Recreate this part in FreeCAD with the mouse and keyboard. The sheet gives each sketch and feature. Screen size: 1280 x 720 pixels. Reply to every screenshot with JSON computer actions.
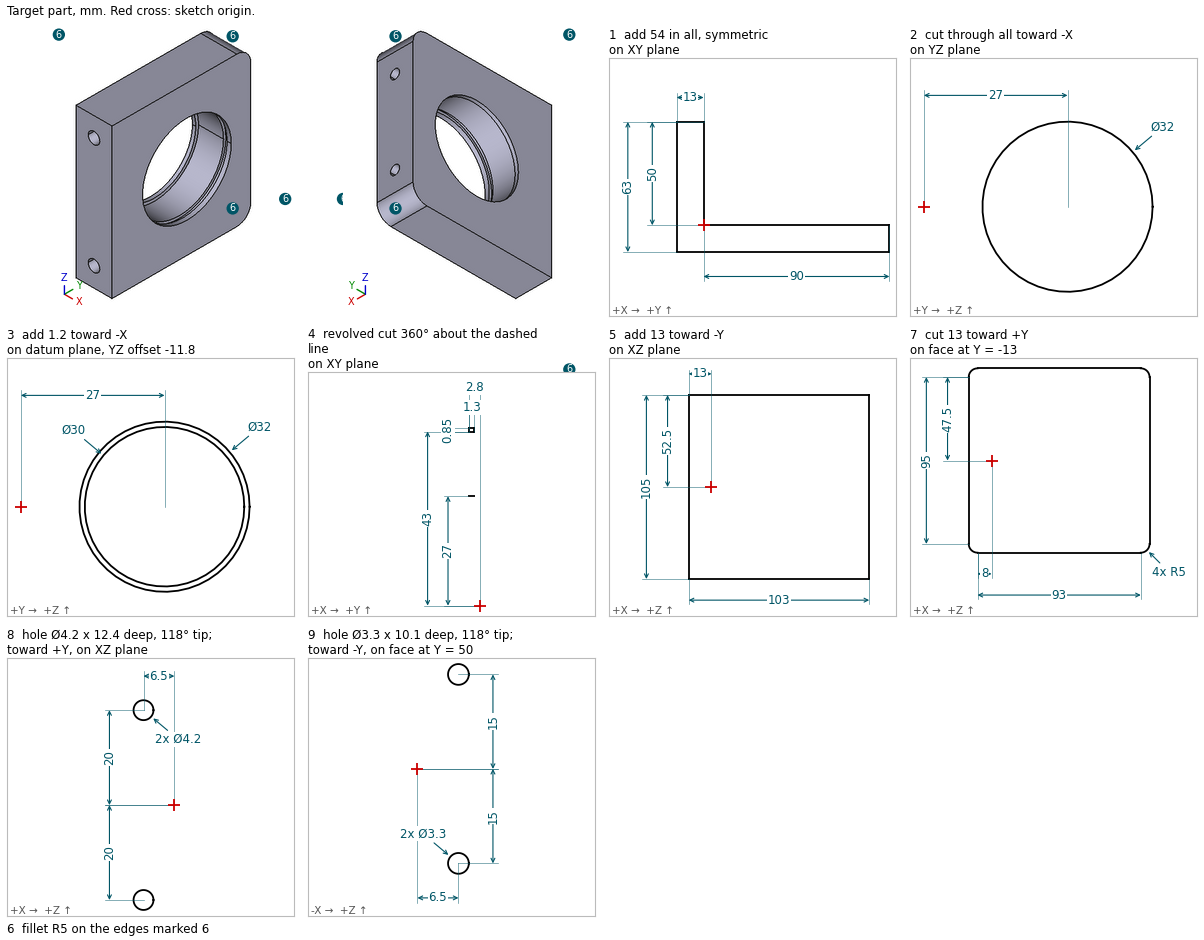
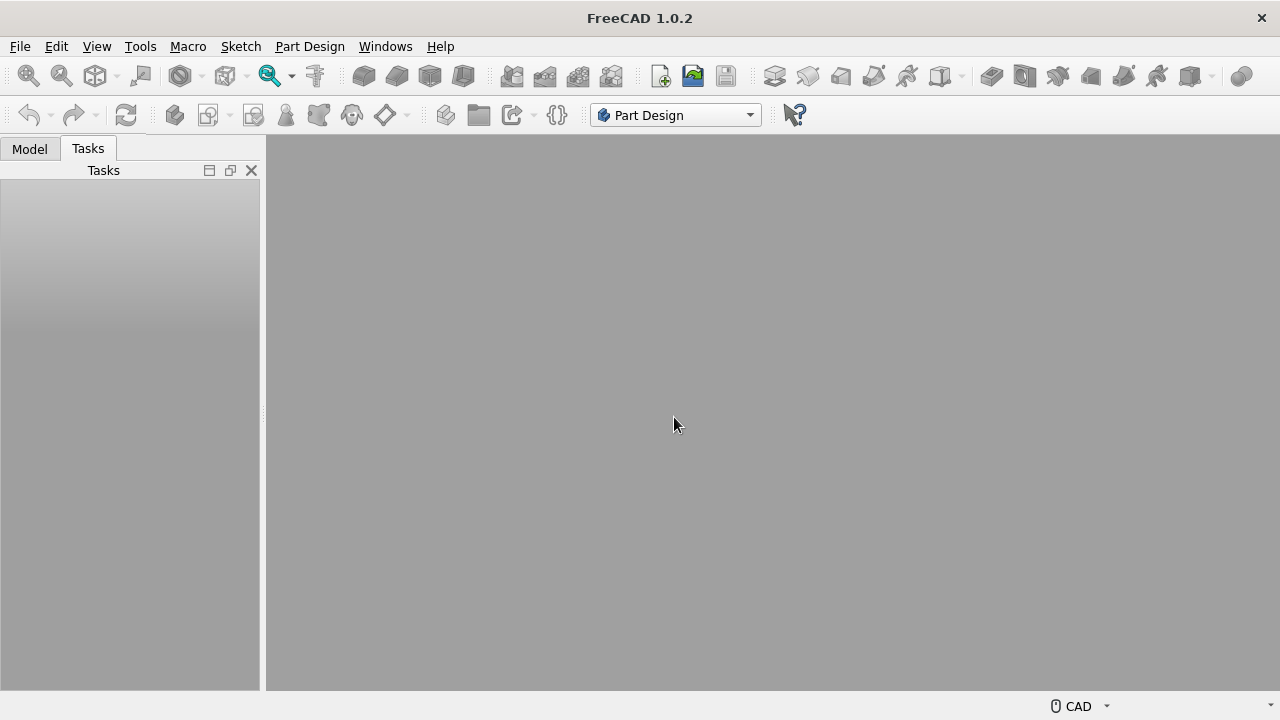
{"action": "left_click", "coordinate": [660, 76]}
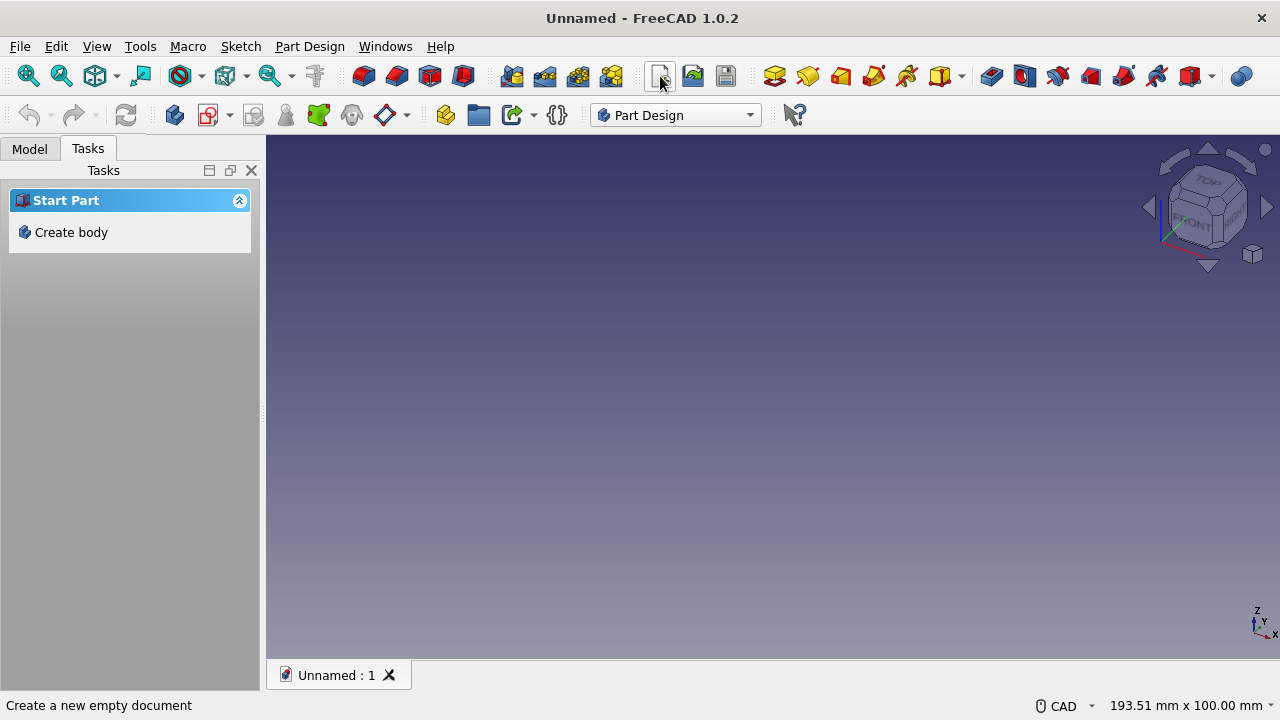
{"action": "left_click", "coordinate": [208, 116]}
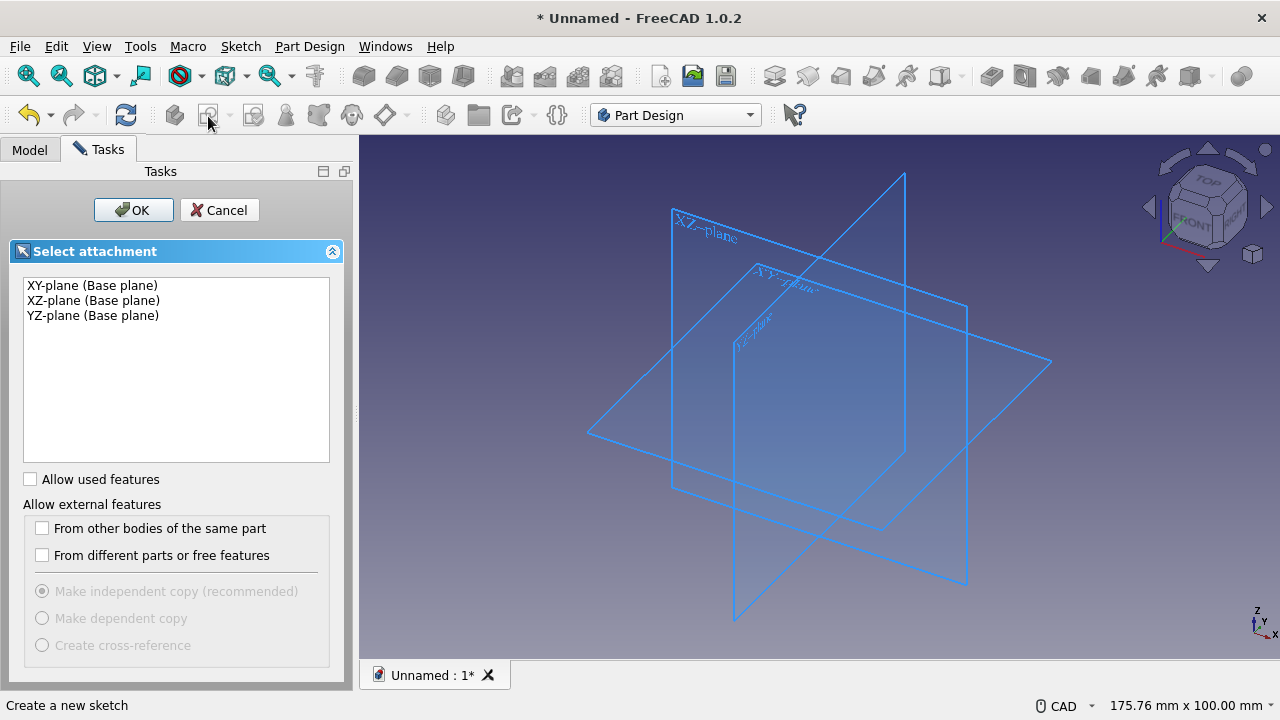
{"action": "left_click", "coordinate": [84, 286]}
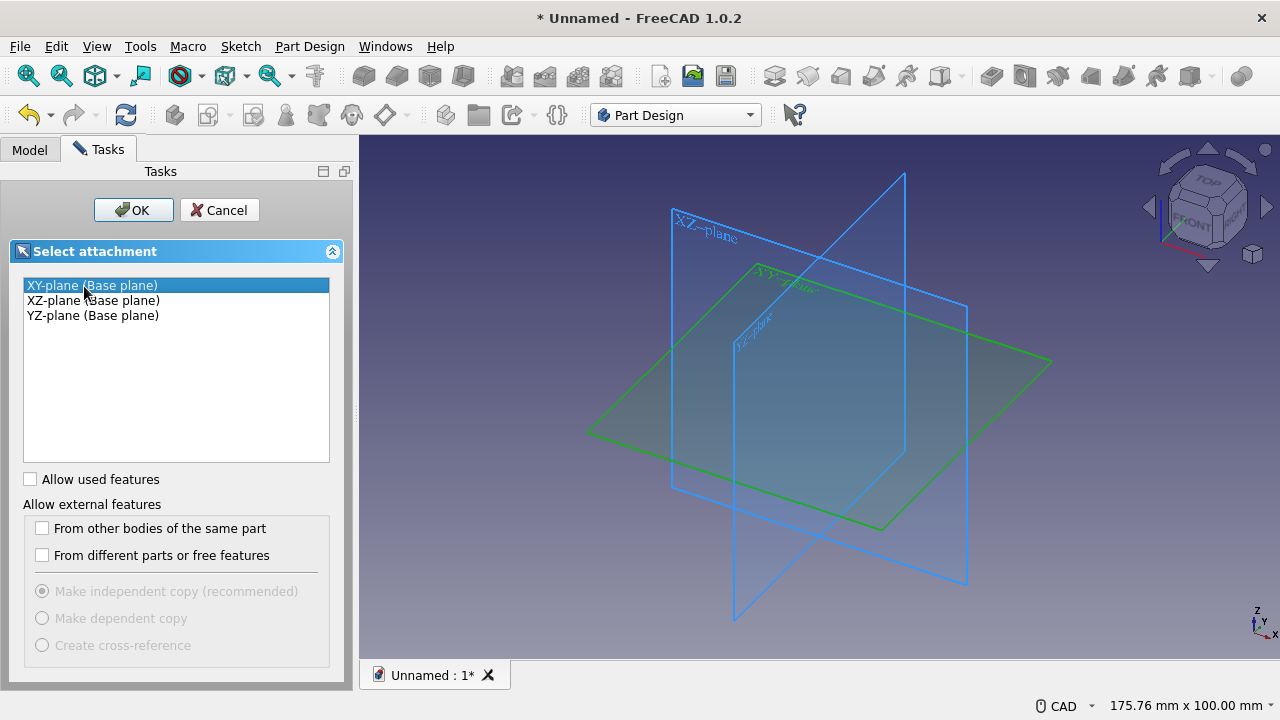
{"action": "left_click", "coordinate": [134, 210]}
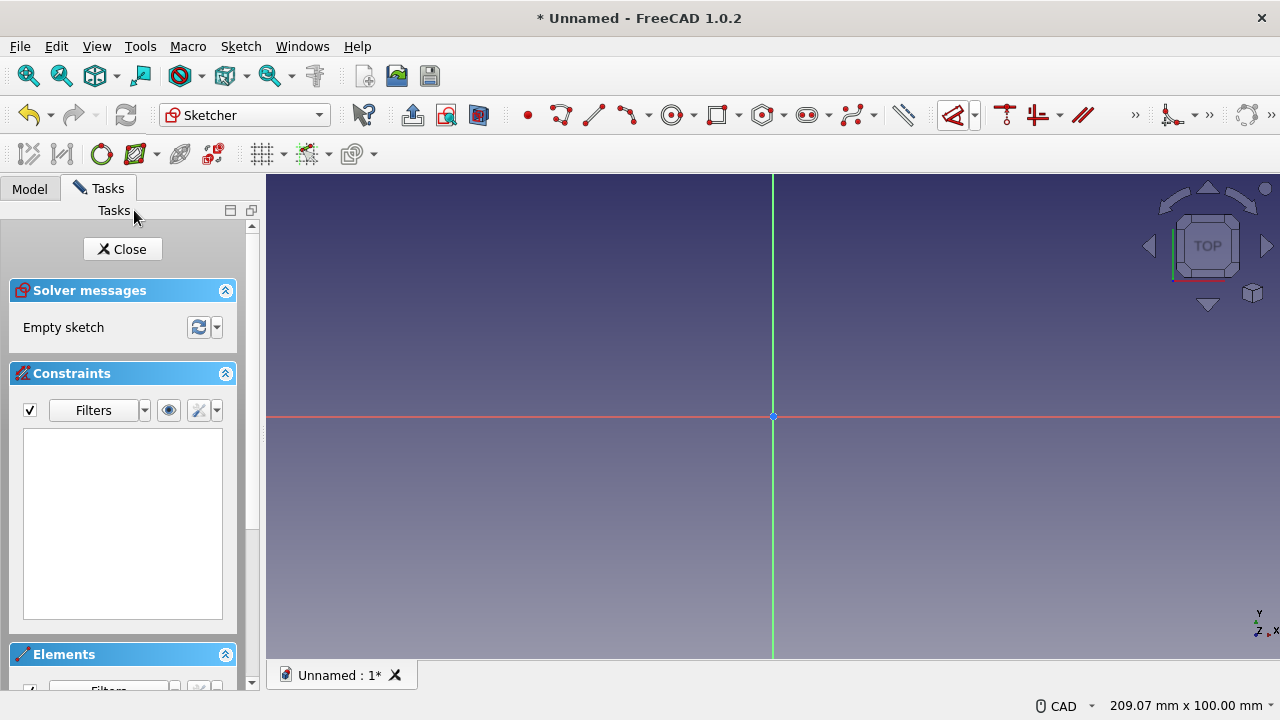
{"action": "scroll", "coordinate": [294, 631], "scroll_direction": "down", "scroll_amount": 1}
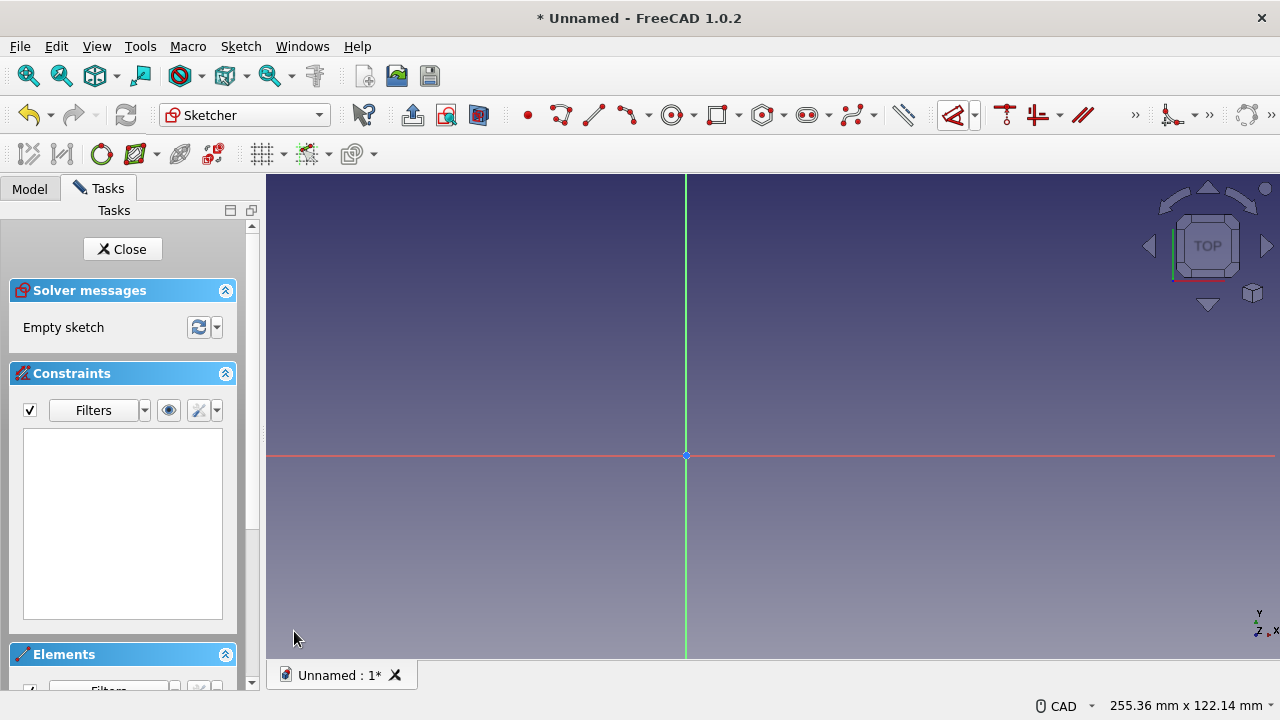
{"action": "left_click", "coordinate": [561, 116]}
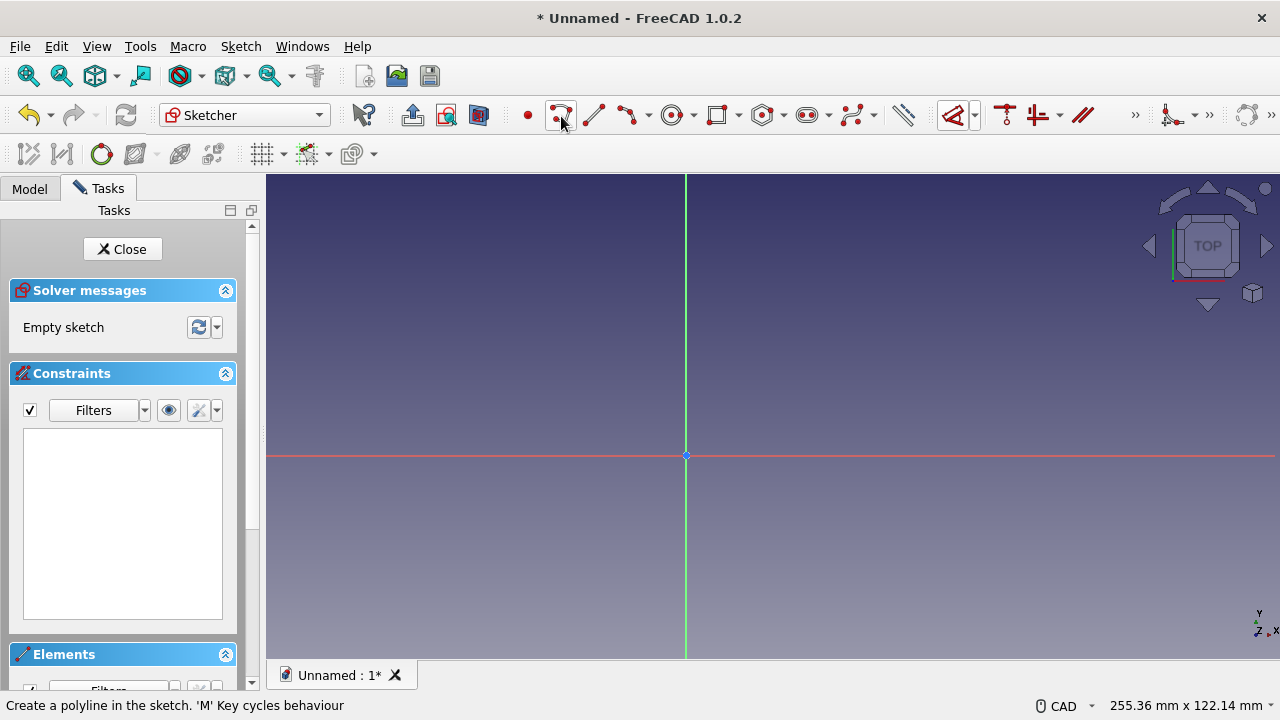
{"action": "left_click", "coordinate": [686, 456]}
{"action": "left_click", "coordinate": [695, 257]}
{"action": "left_click", "coordinate": [635, 257]}
{"action": "left_click", "coordinate": [635, 507]}
{"action": "left_click", "coordinate": [1044, 507]}
{"action": "left_click", "coordinate": [1044, 447]}
{"action": "left_click", "coordinate": [686, 456]}
{"action": "key", "text": "Escape"}
{"action": "key", "text": "Escape"}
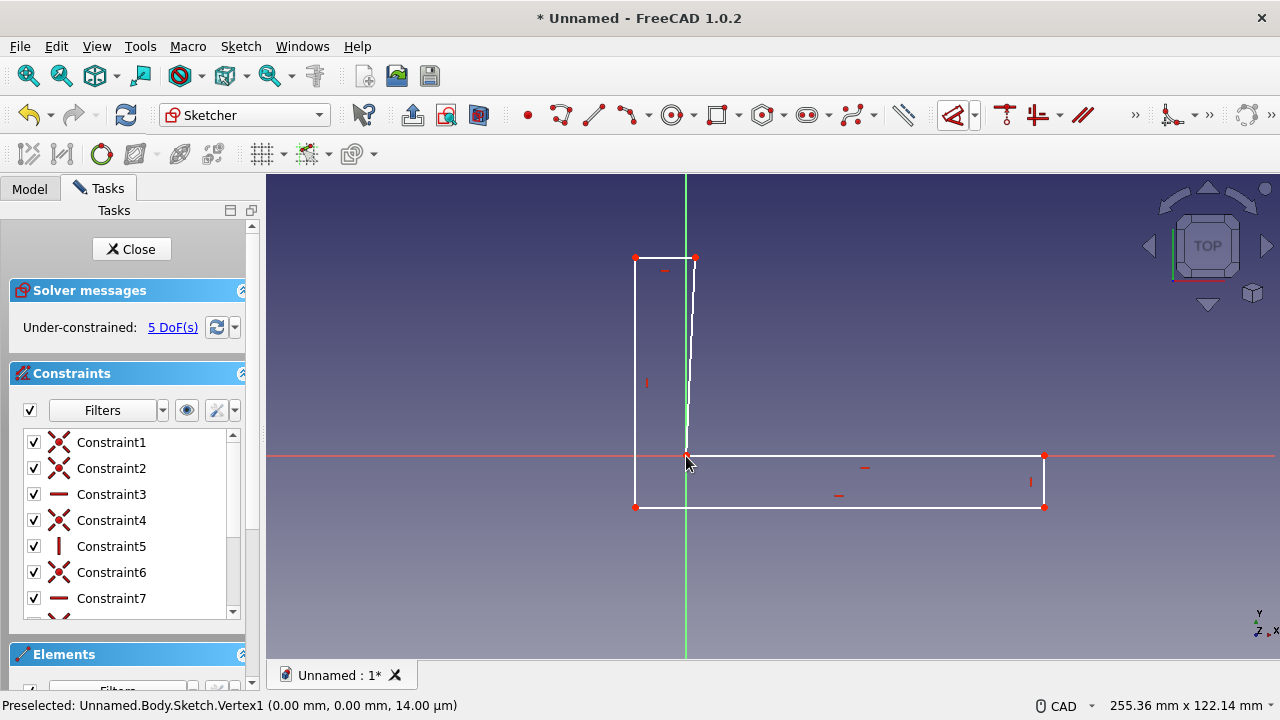
{"action": "left_click", "coordinate": [689, 396]}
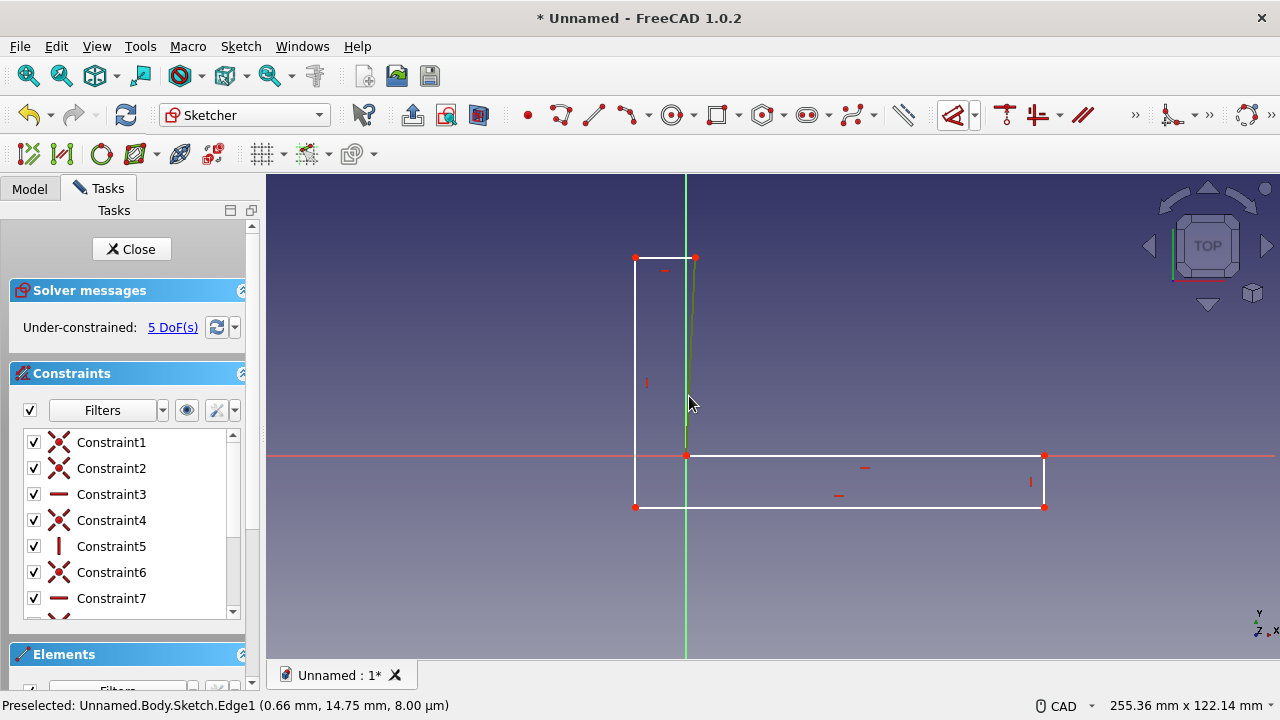
{"action": "left_click", "coordinate": [1060, 116]}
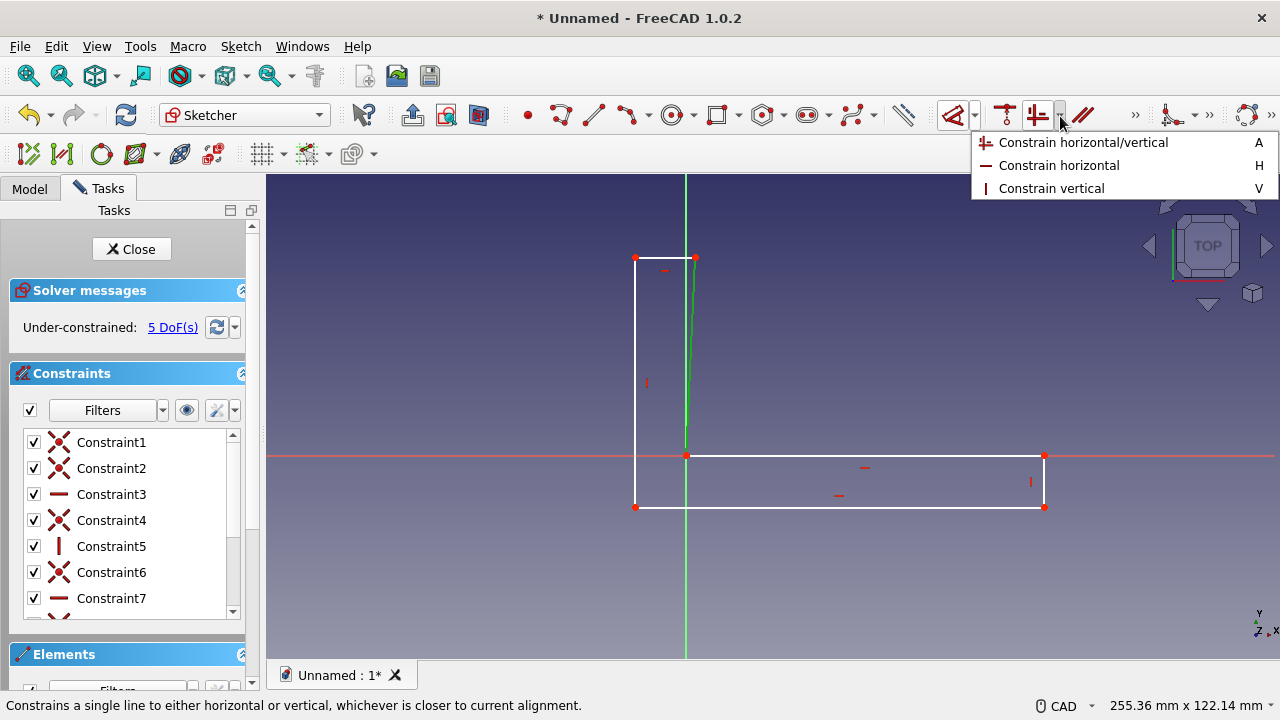
{"action": "left_click", "coordinate": [1125, 188]}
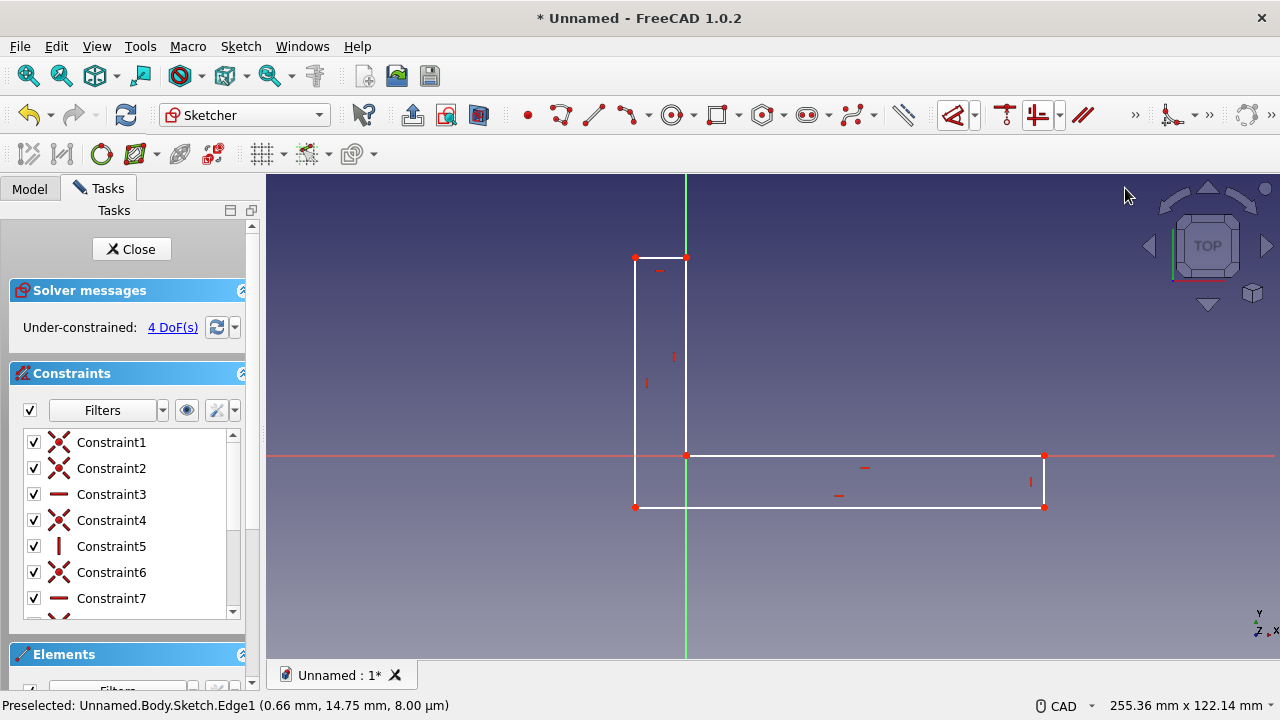
{"action": "left_click", "coordinate": [686, 396]}